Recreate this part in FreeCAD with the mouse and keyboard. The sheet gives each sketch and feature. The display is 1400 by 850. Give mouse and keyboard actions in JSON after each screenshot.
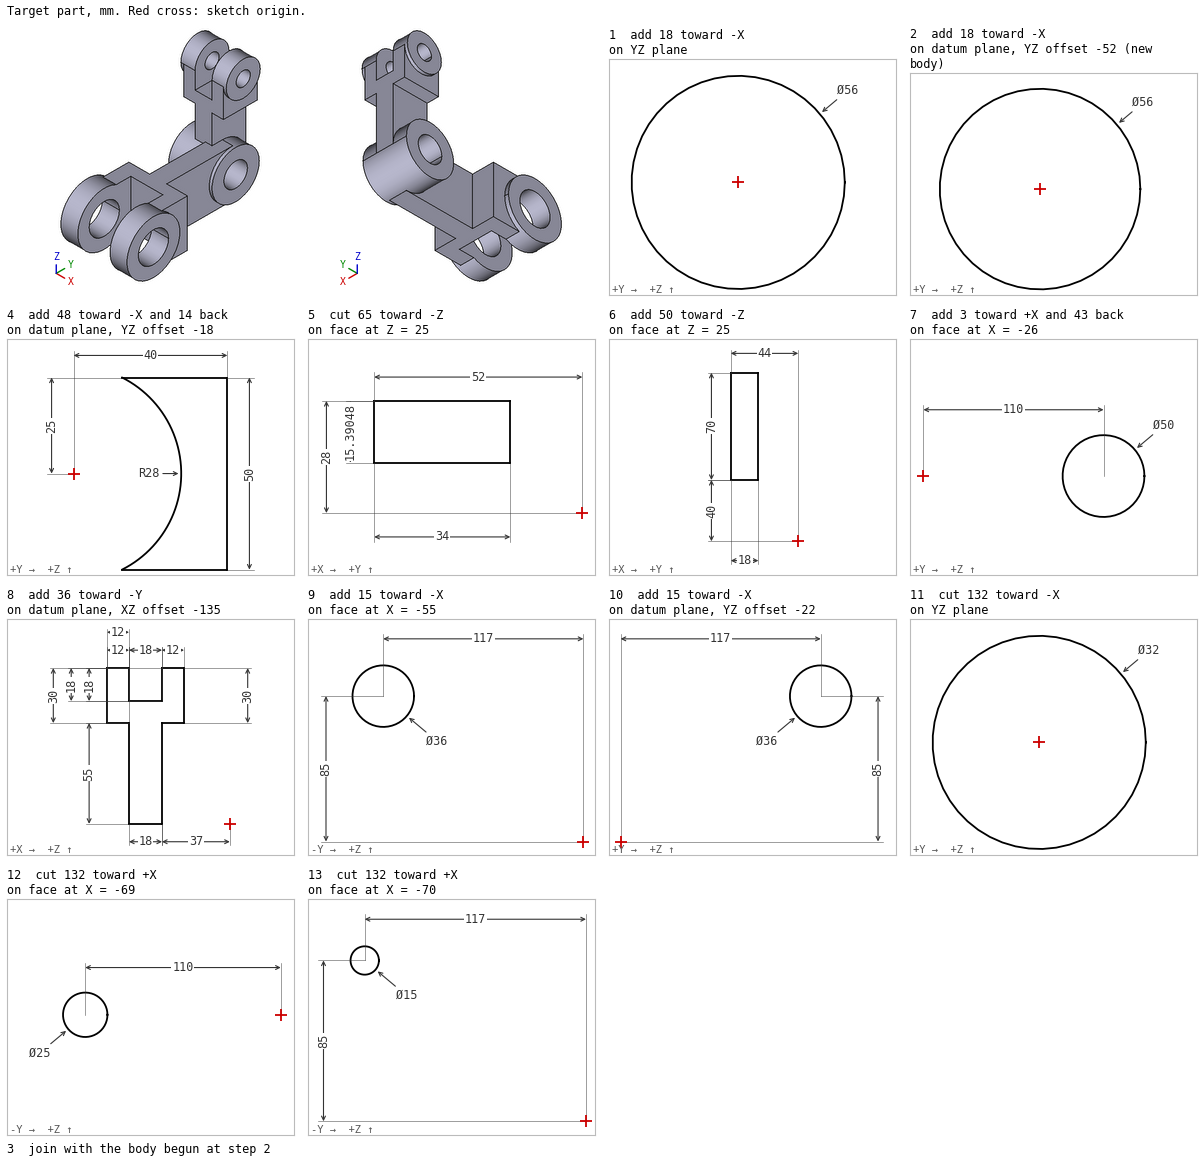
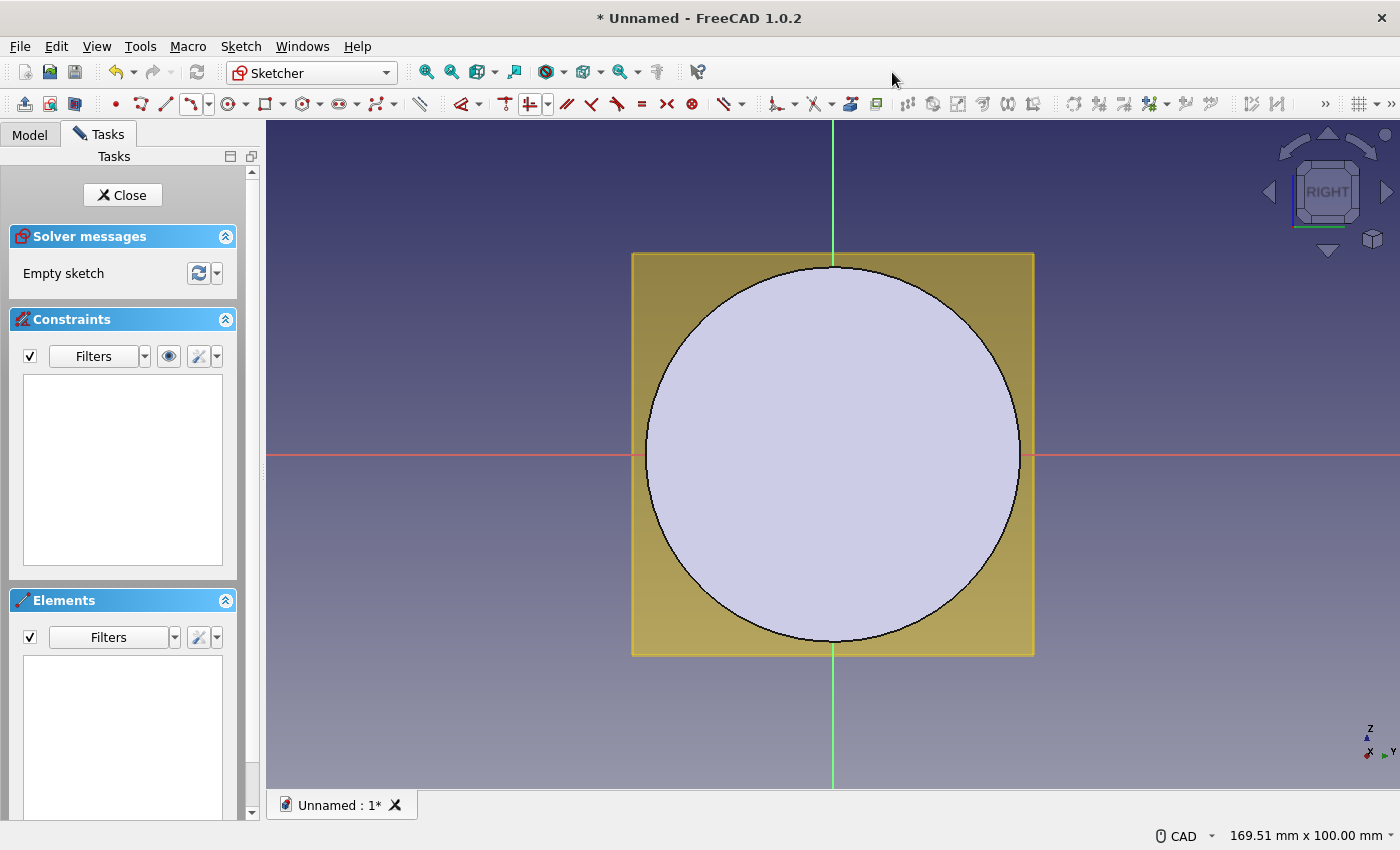
{"action": "key", "text": "g c"}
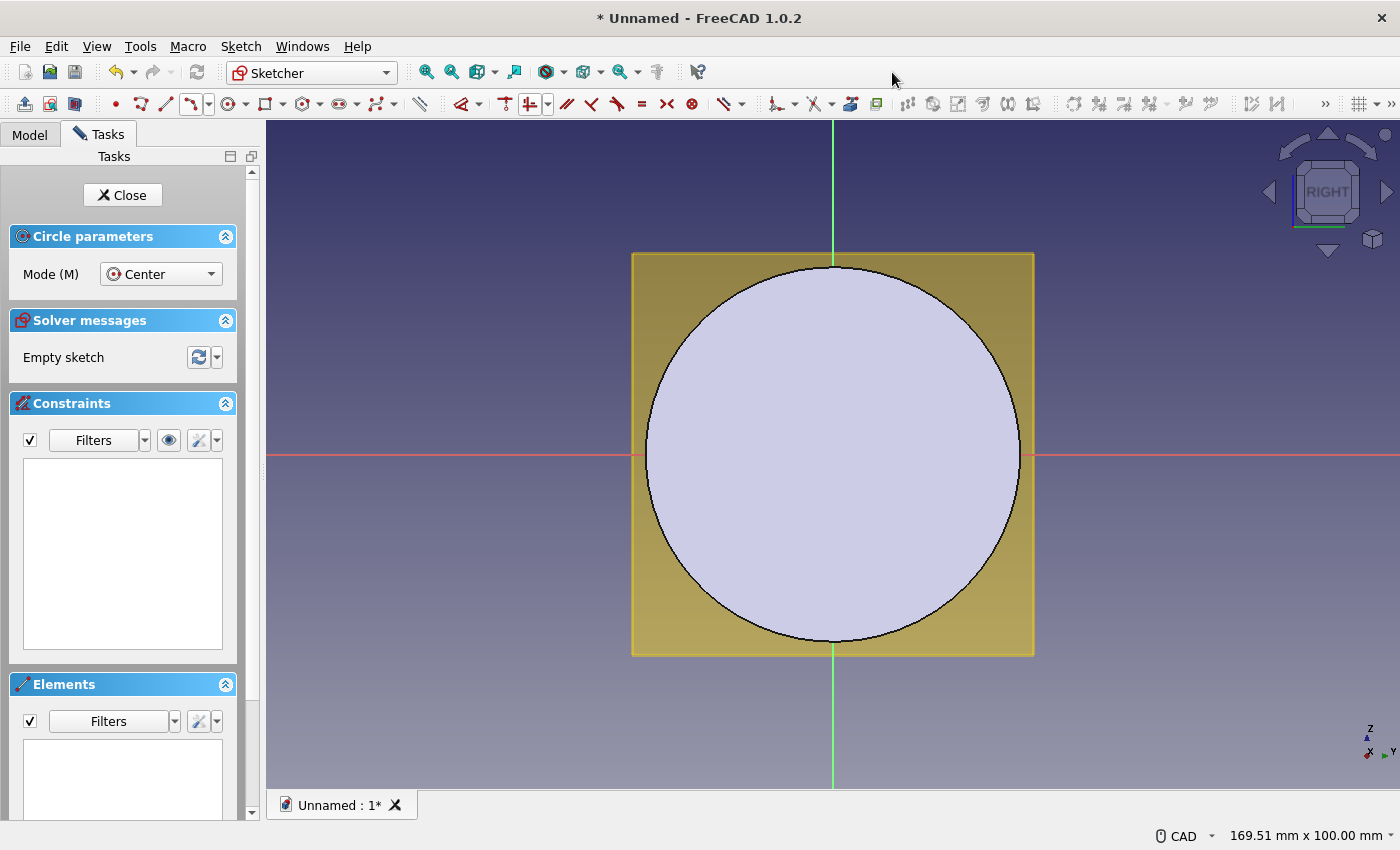
{"action": "left_click", "coordinate": [833, 454]}
{"action": "left_click", "coordinate": [965, 322]}
{"action": "key", "text": "Escape"}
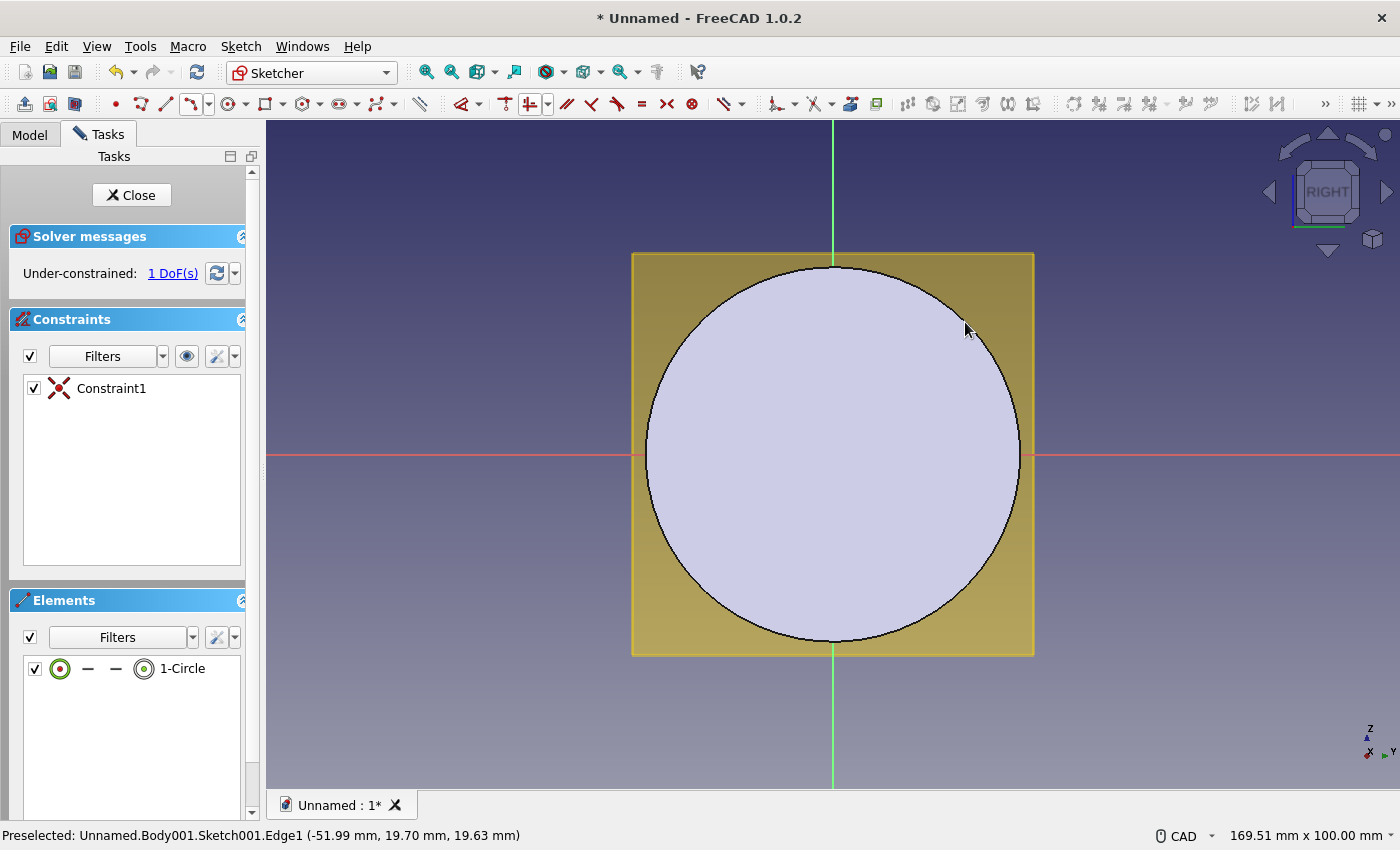
{"action": "left_click", "coordinate": [964, 322]}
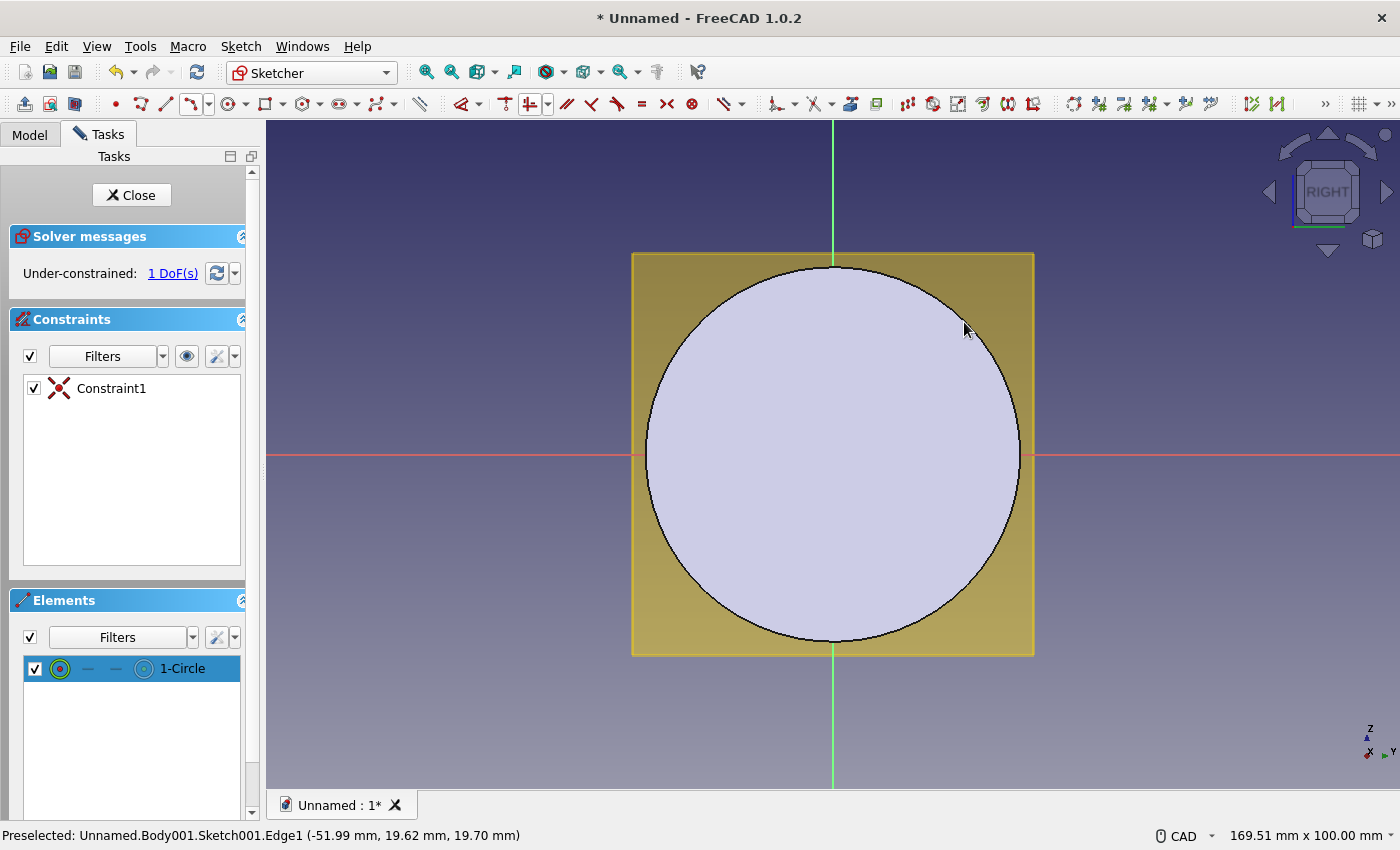
{"action": "key", "text": "k o"}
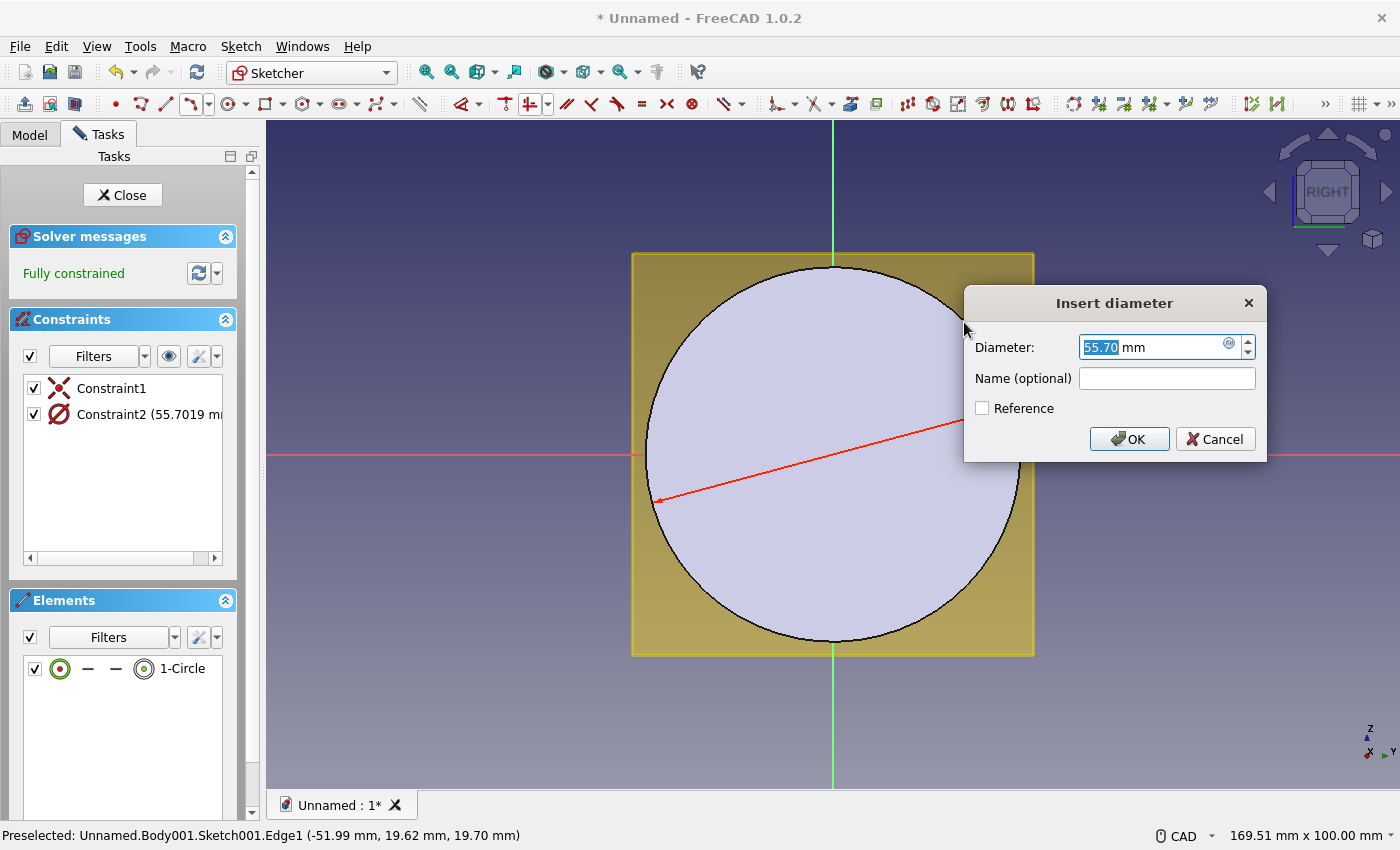
{"action": "type", "text": "56"}
{"action": "key", "text": "Return"}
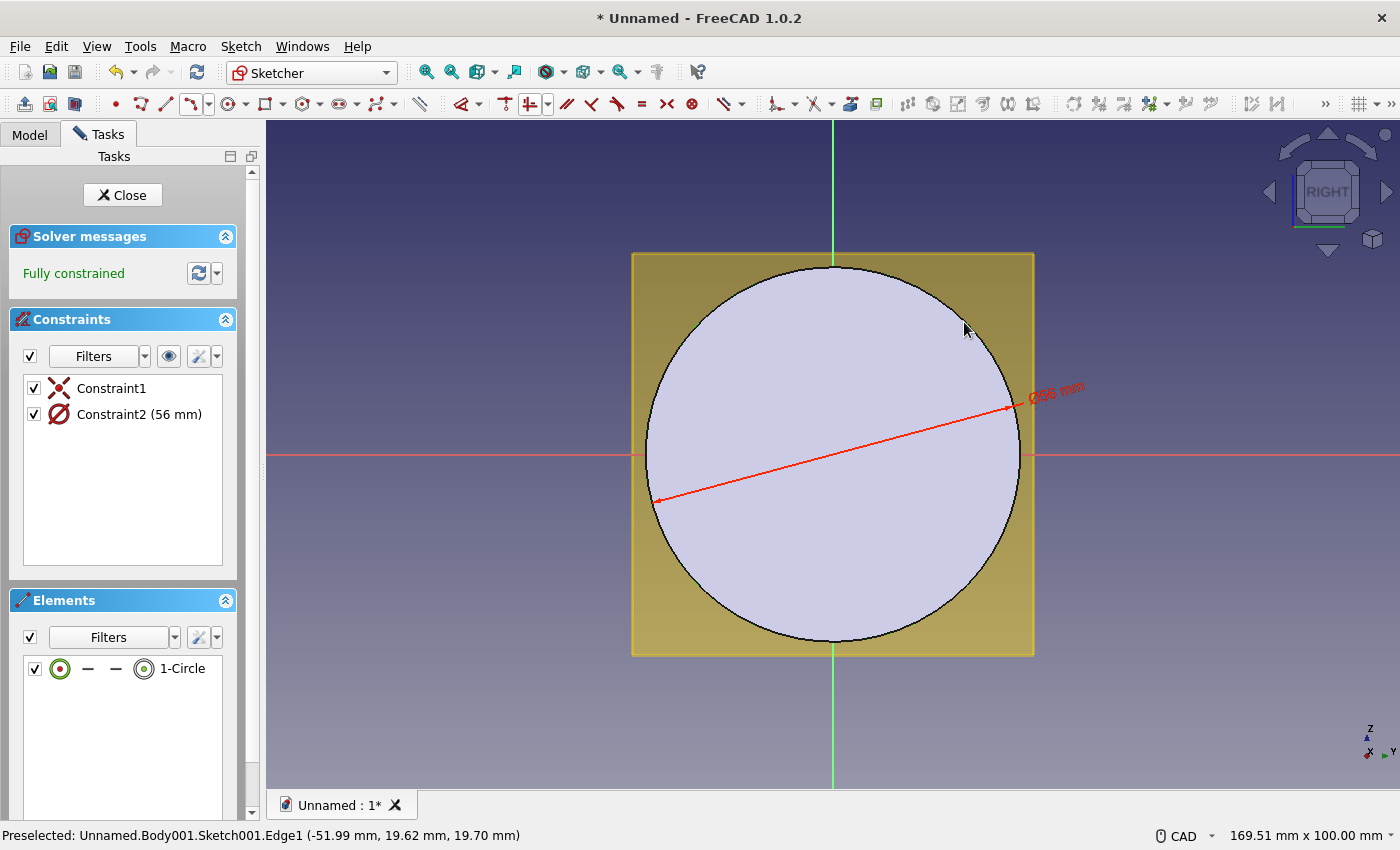
{"action": "left_click", "coordinate": [123, 195]}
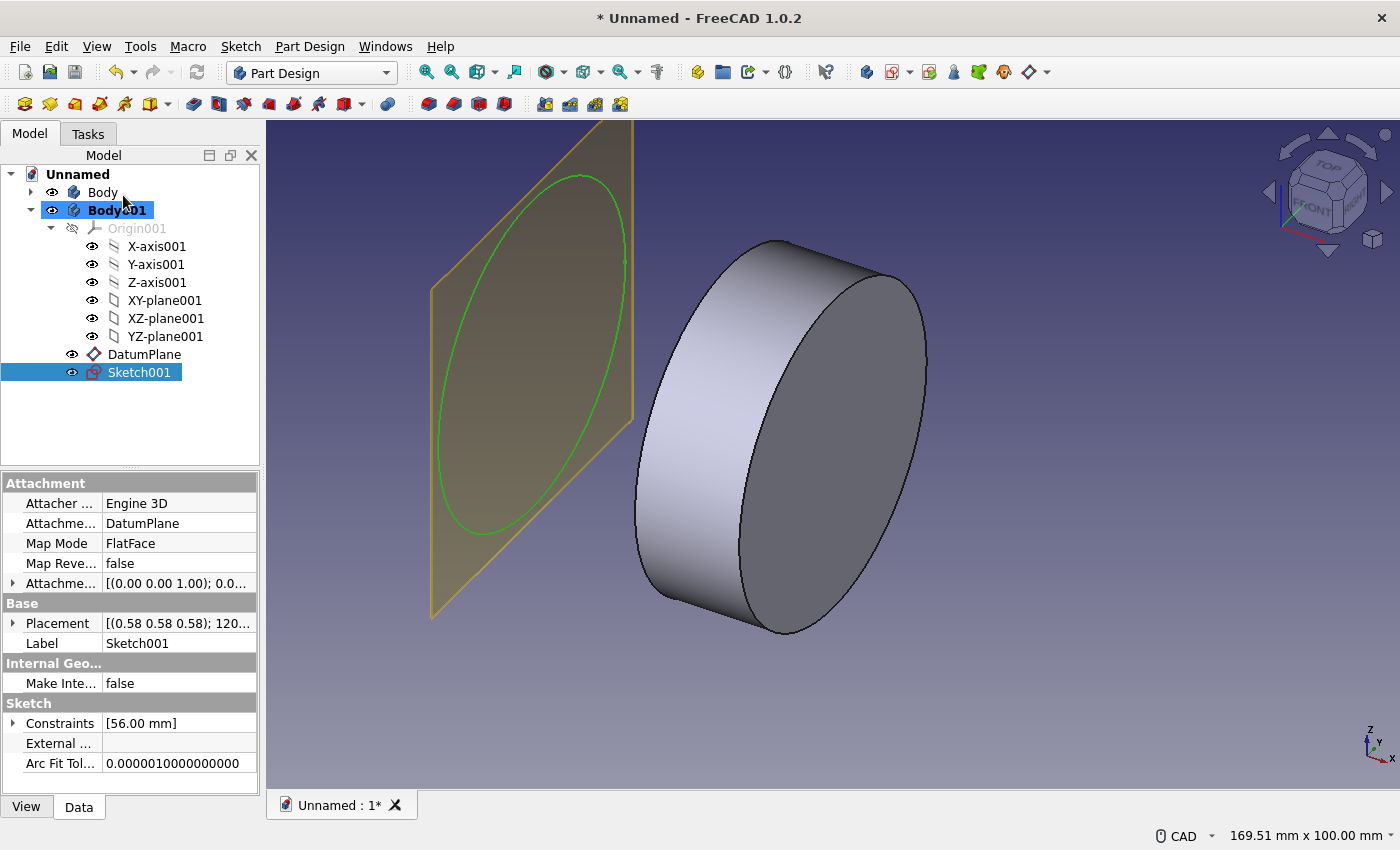
{"action": "left_click", "coordinate": [25, 104]}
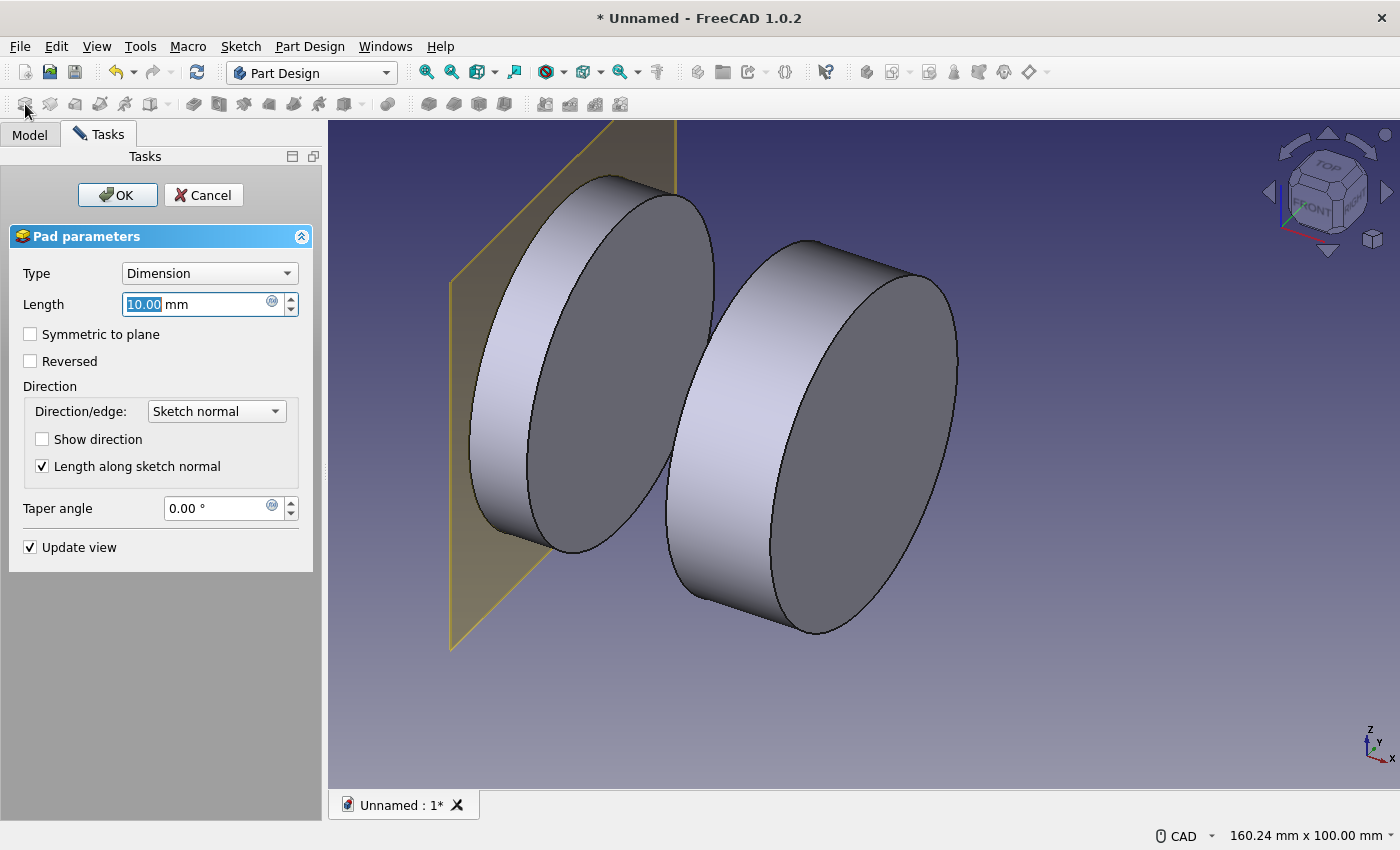
{"action": "type", "text": "18"}
{"action": "key", "text": "Tab"}